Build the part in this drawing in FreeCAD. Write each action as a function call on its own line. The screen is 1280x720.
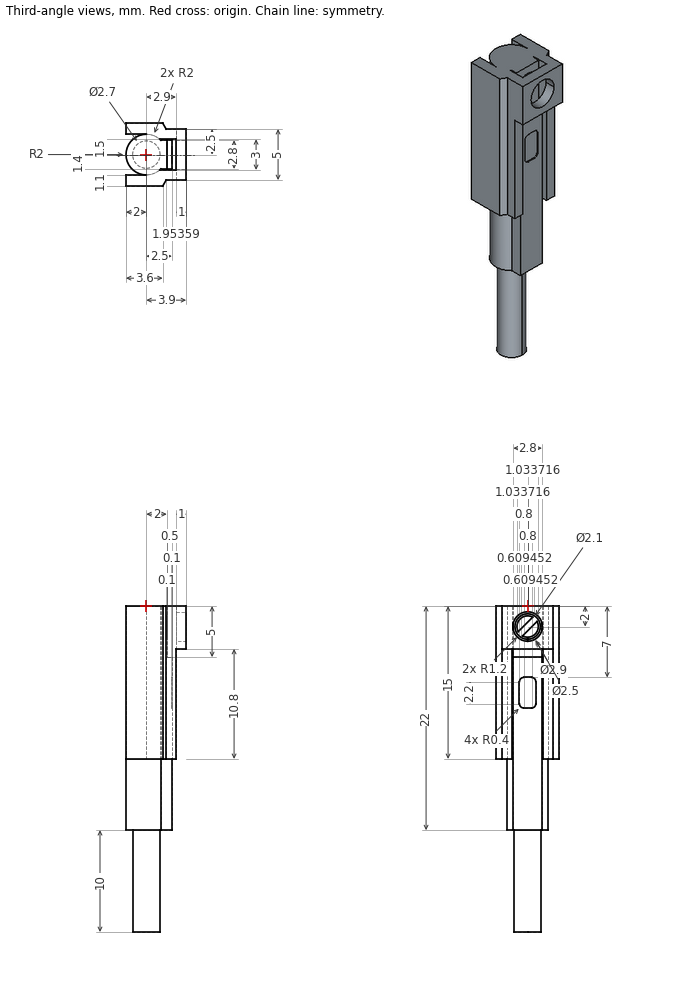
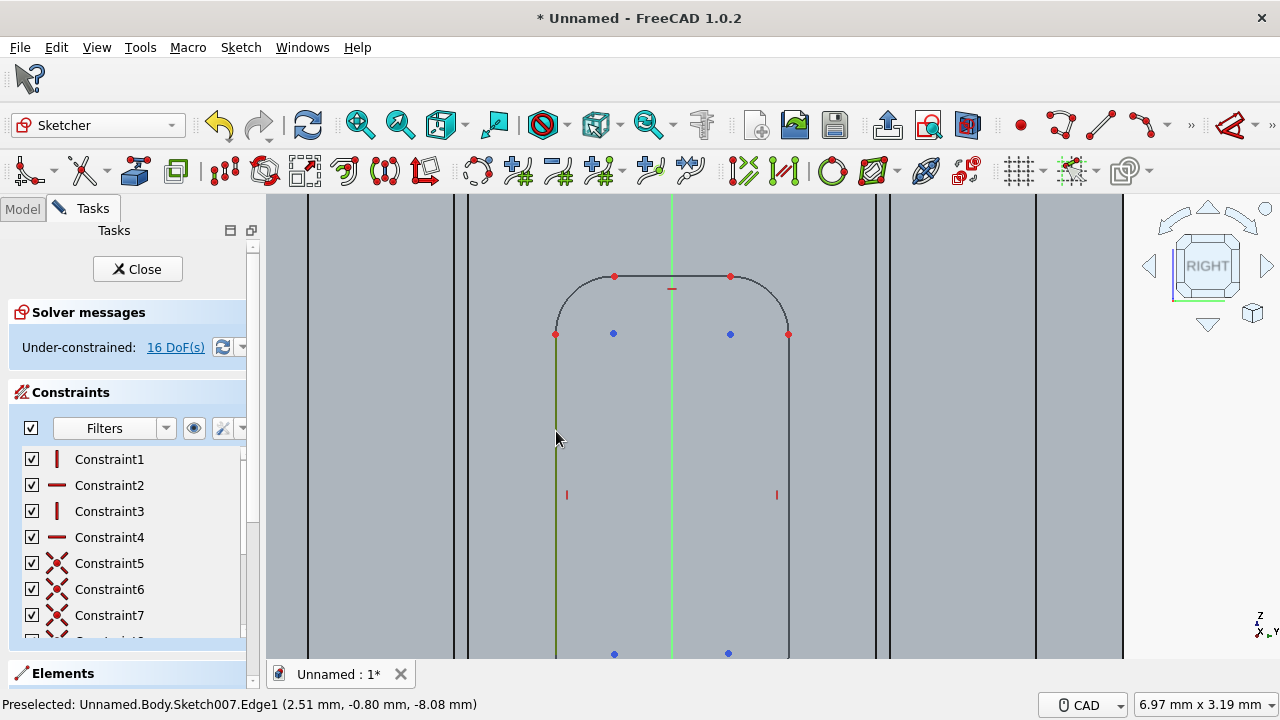
scroll(771, 291, down, 2)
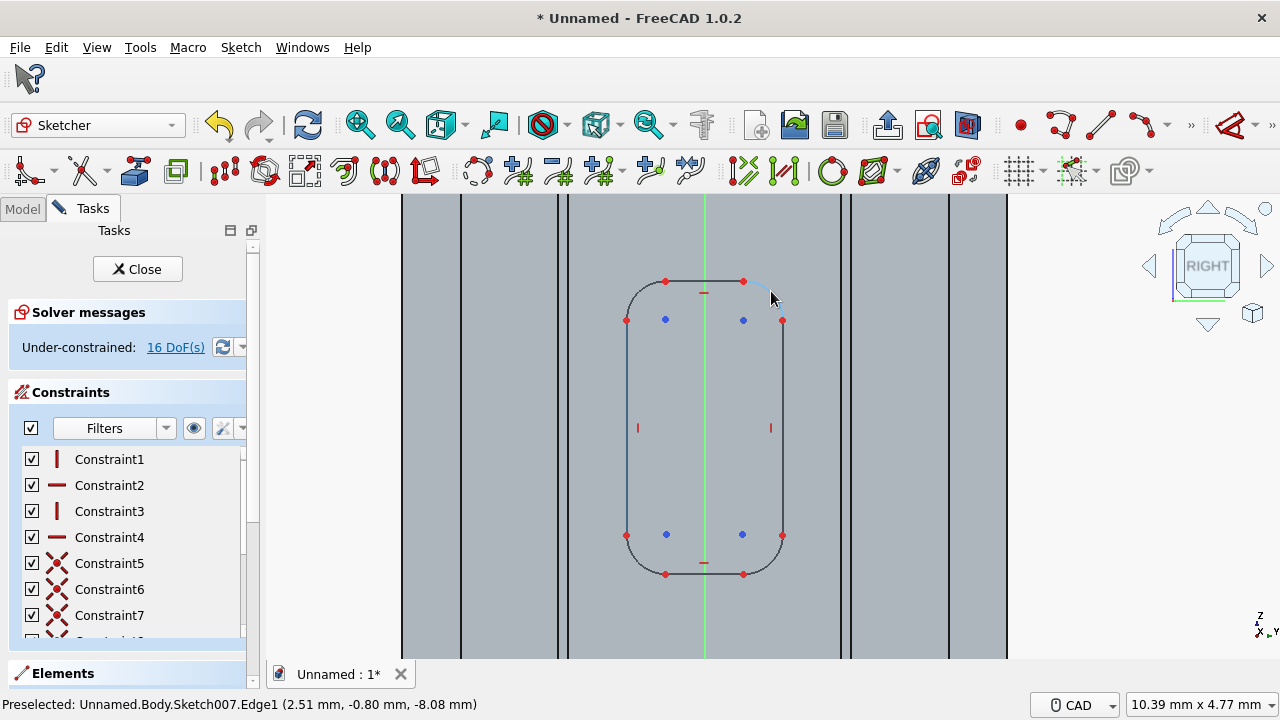
click(631, 553)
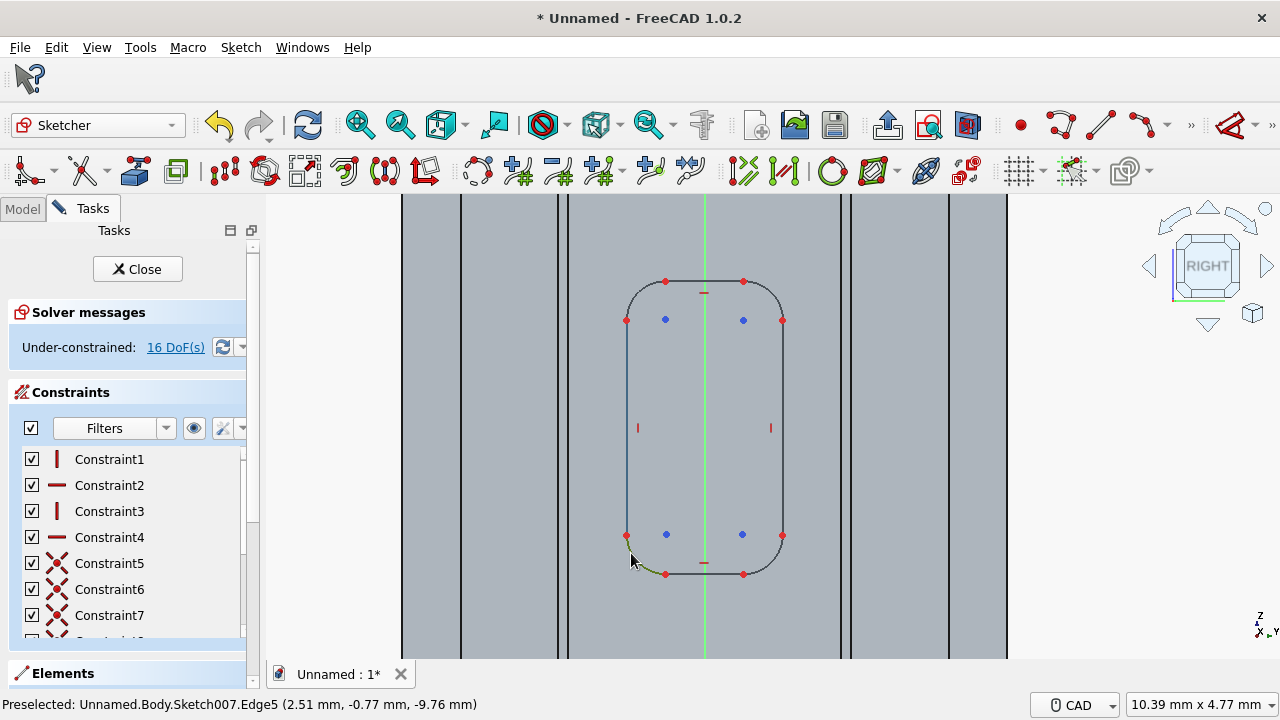
key(t)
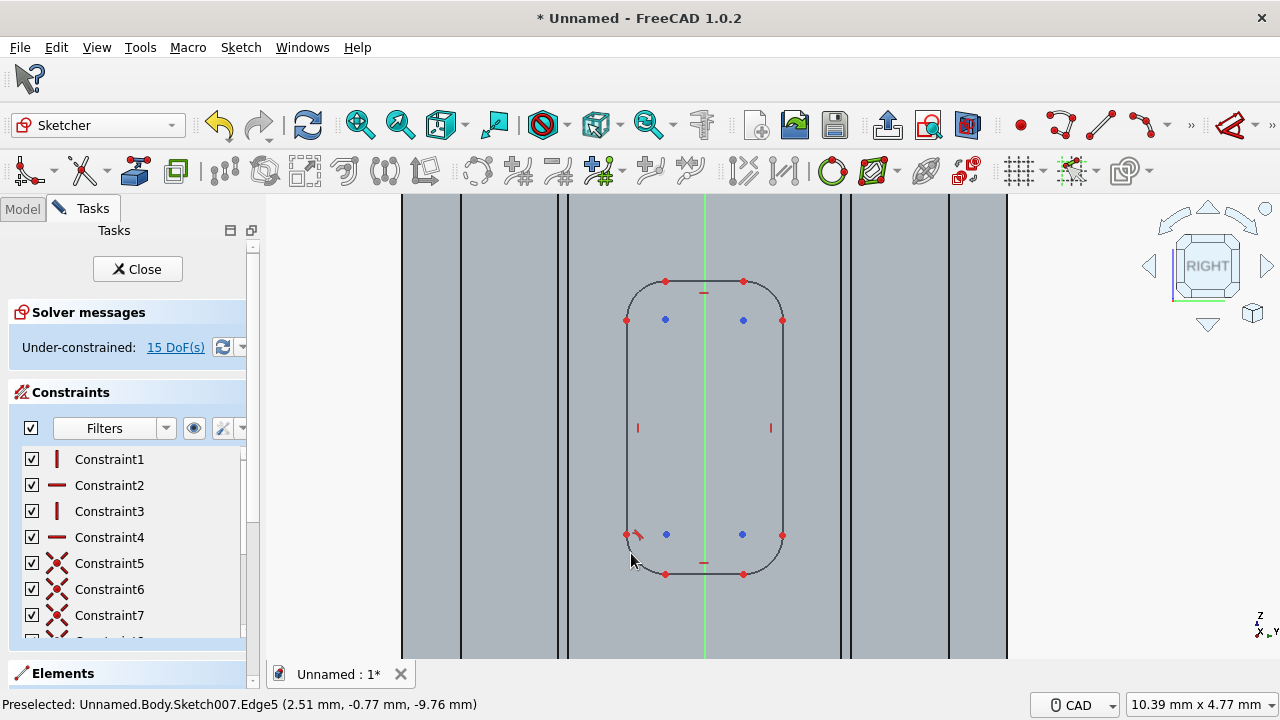
click(627, 385)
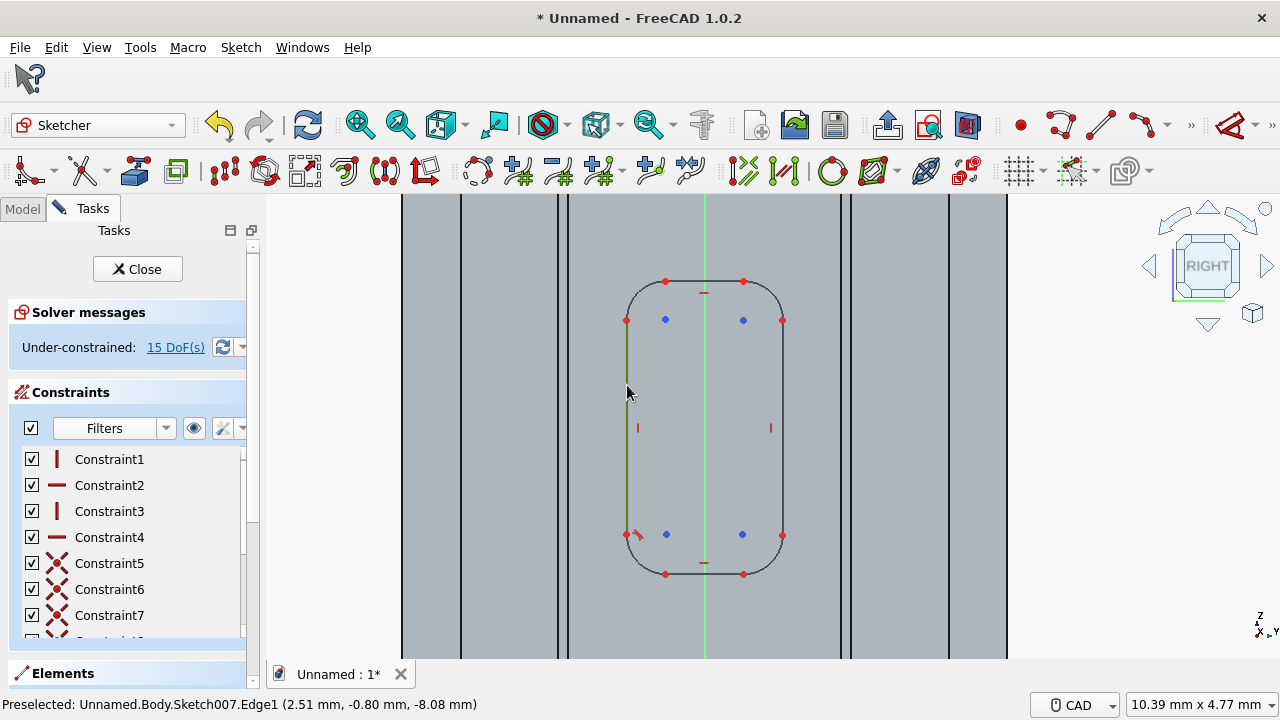
click(648, 285)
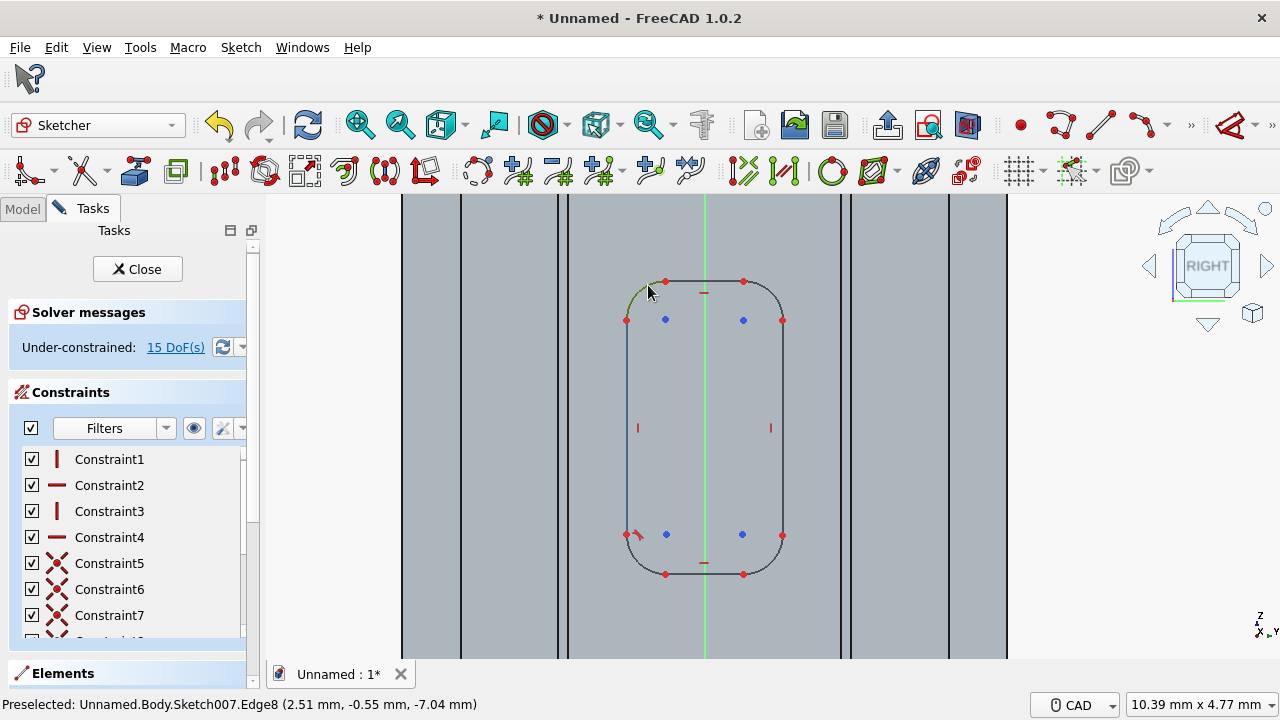
key(t)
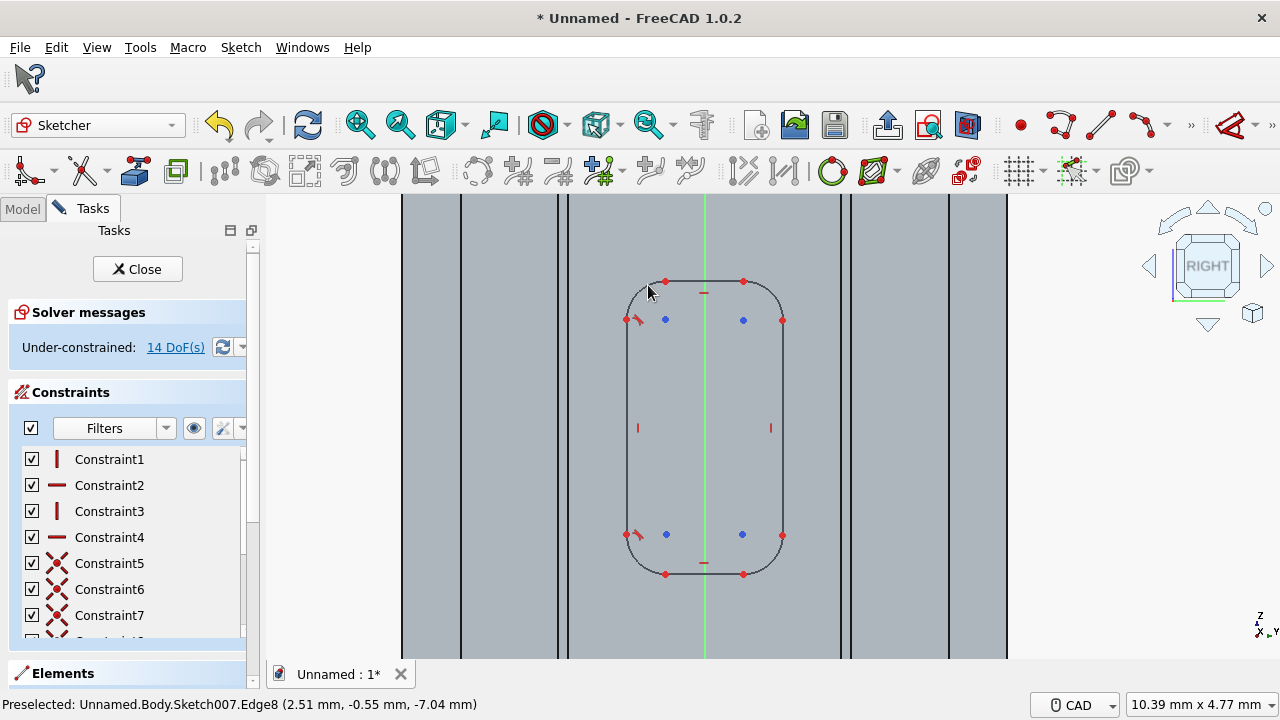
click(689, 574)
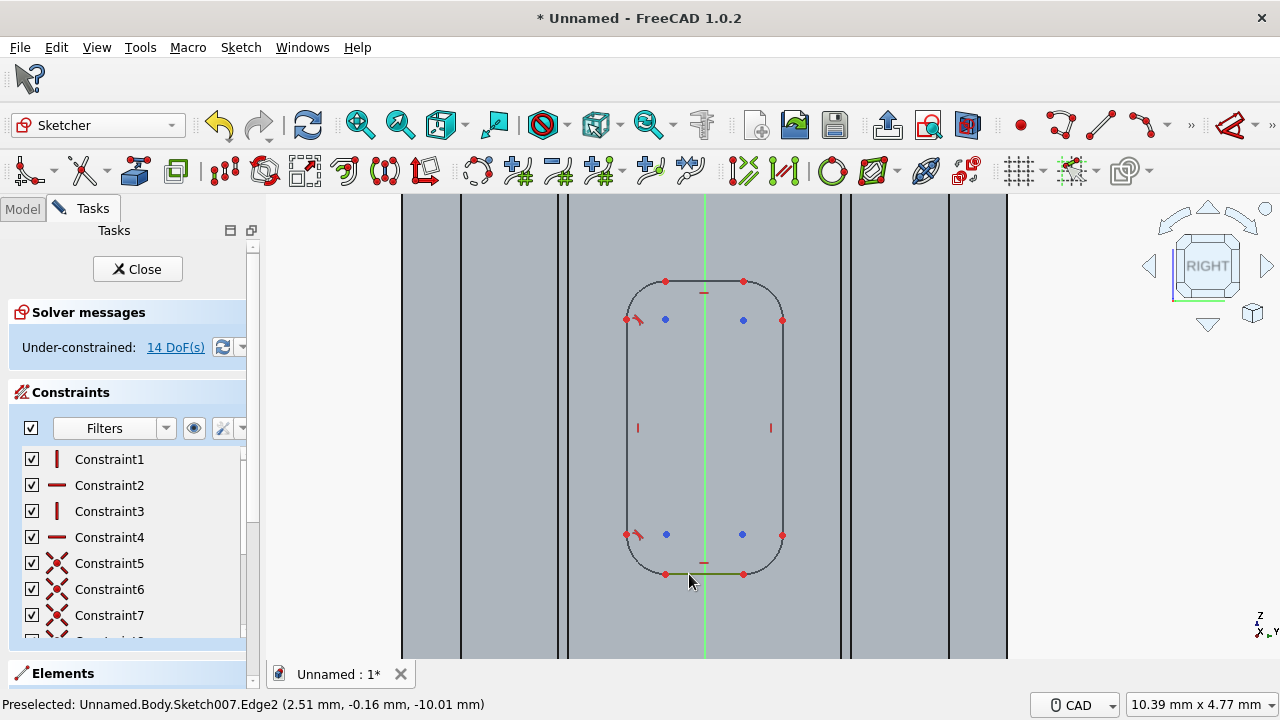
click(631, 553)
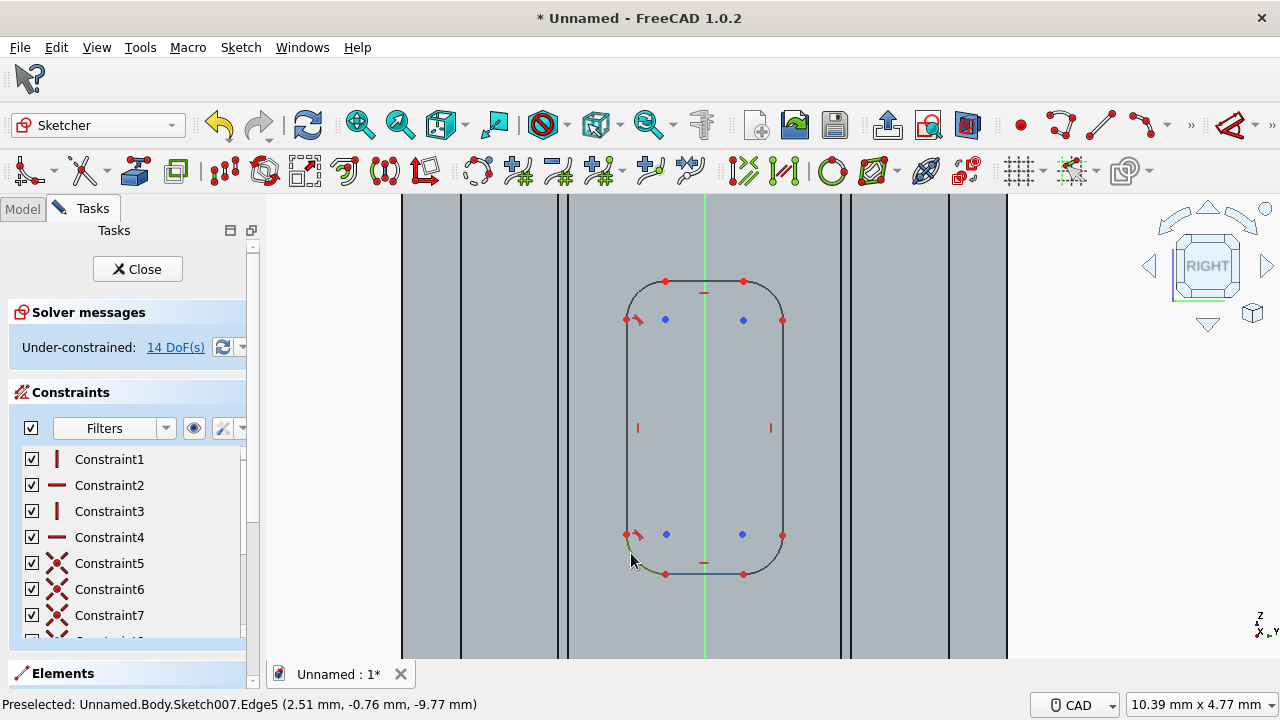
key(t)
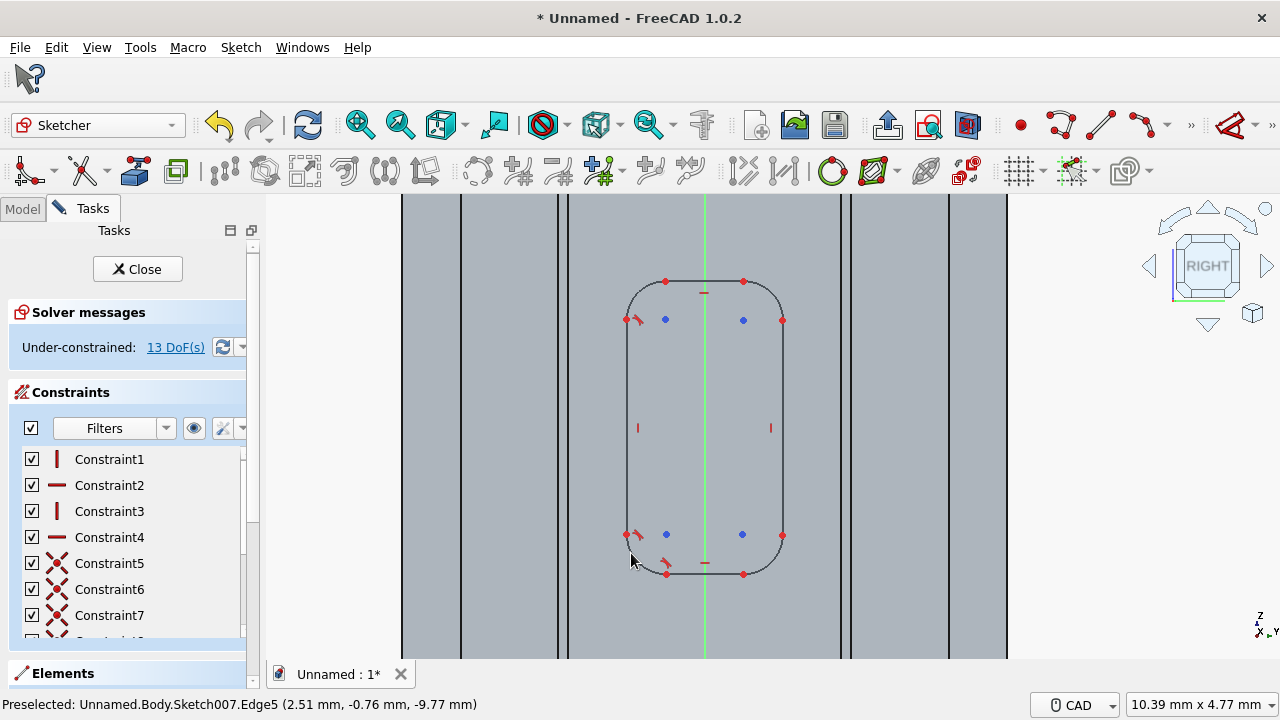
click(690, 574)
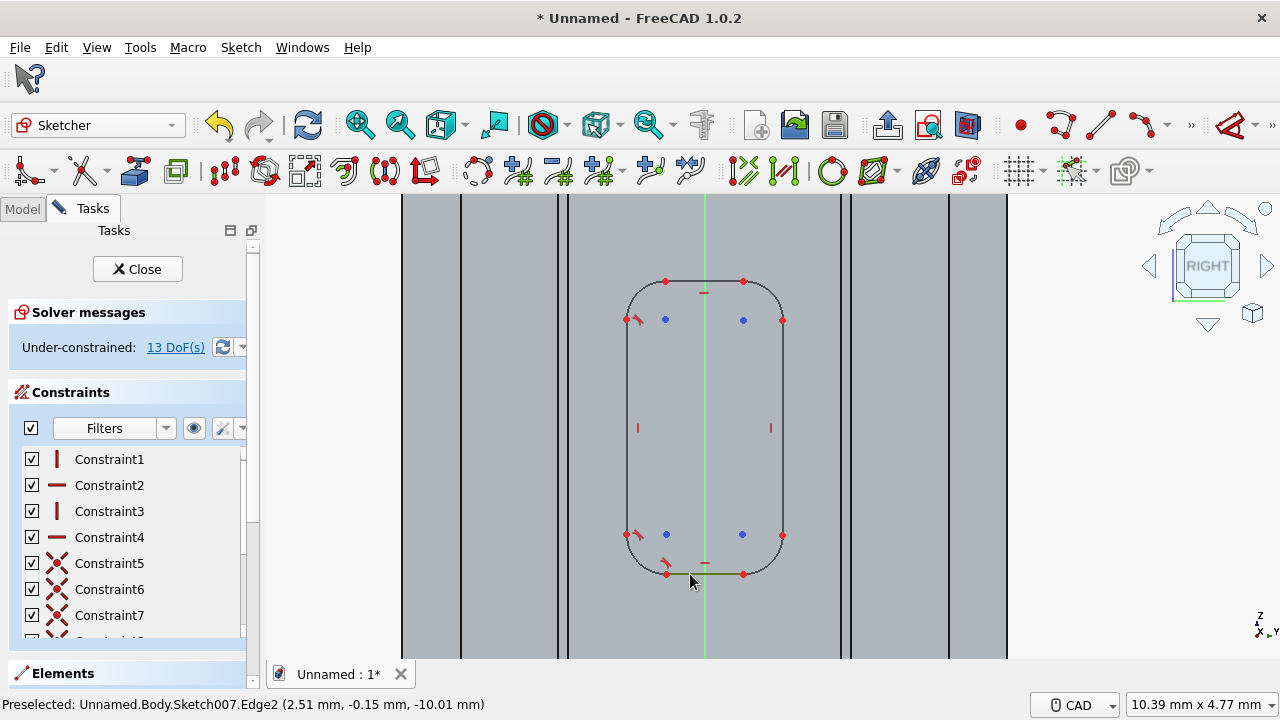
click(761, 570)